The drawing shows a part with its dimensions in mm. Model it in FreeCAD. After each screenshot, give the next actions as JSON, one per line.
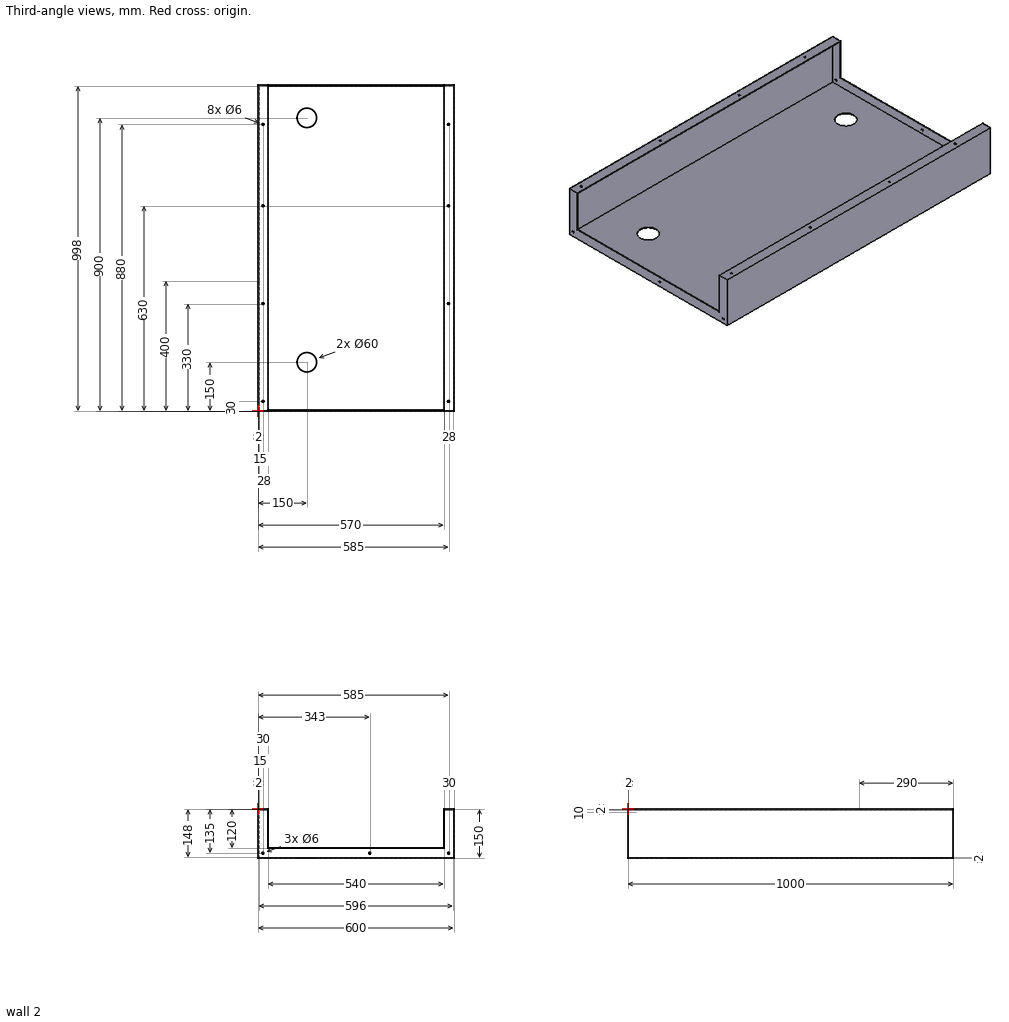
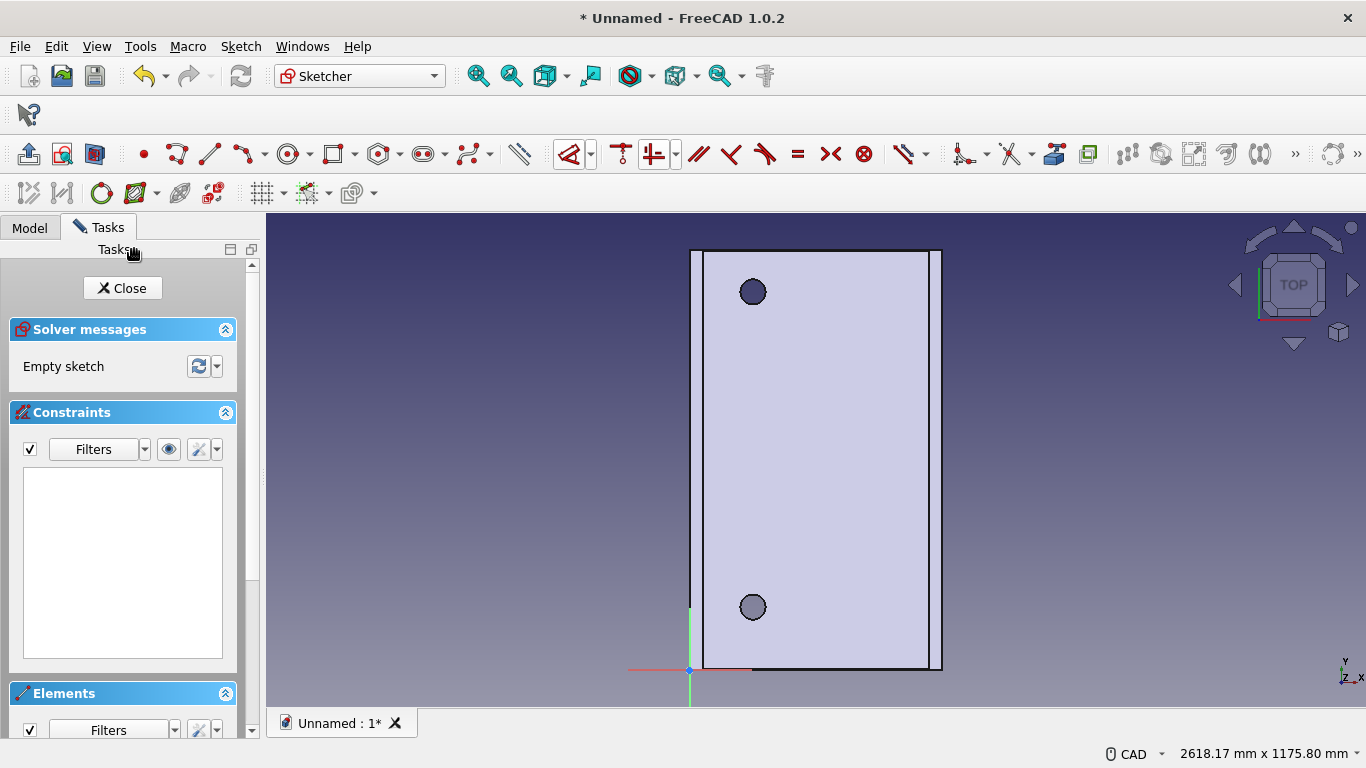
{"action": "scroll", "coordinate": [449, 349], "scroll_direction": "down", "scroll_amount": 1}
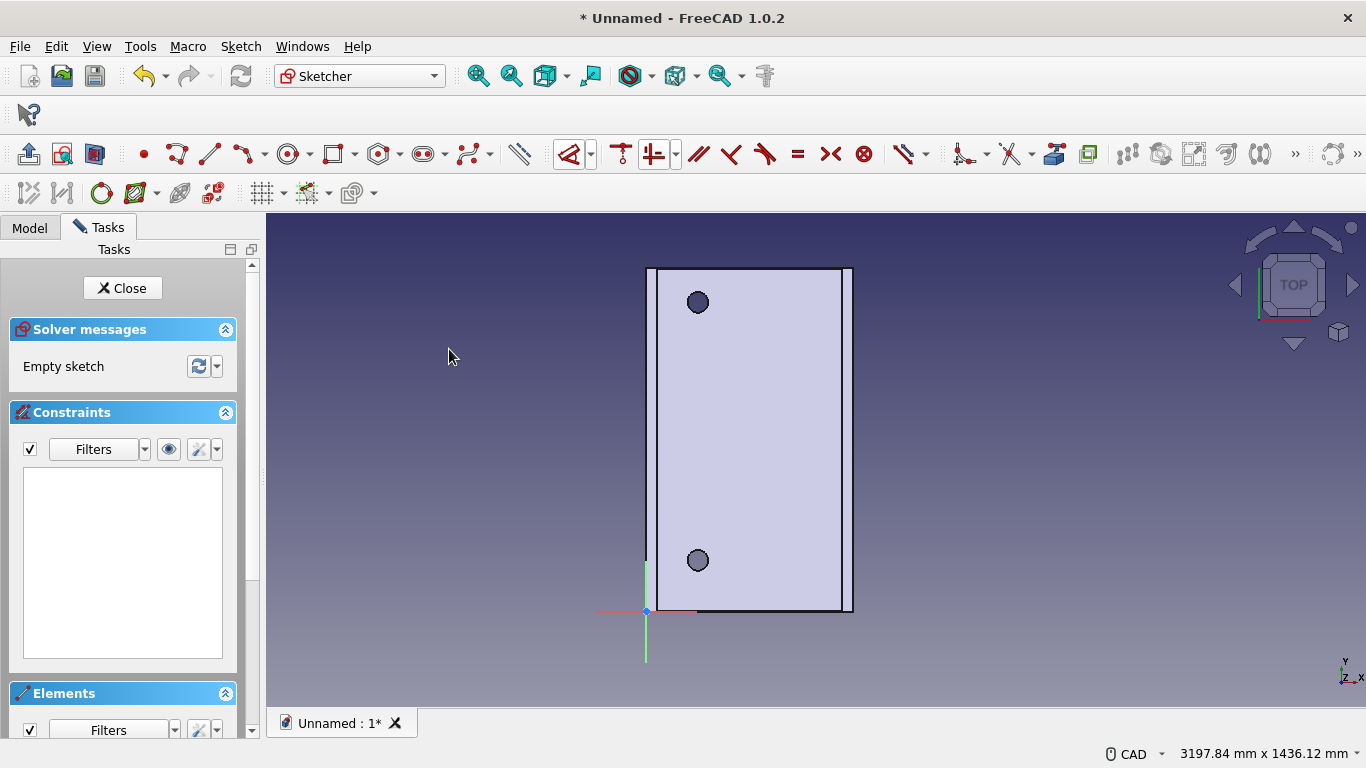
{"action": "left_click", "coordinate": [288, 154]}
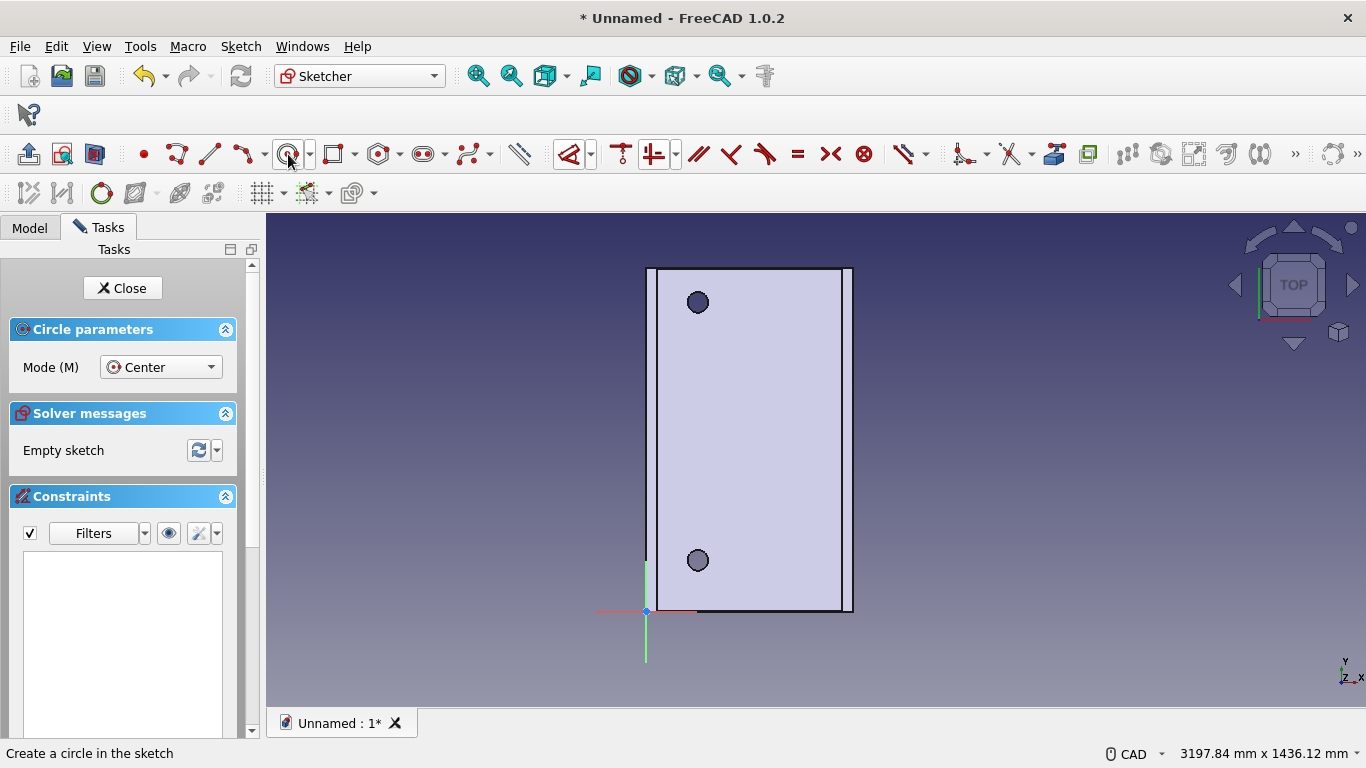
{"action": "scroll", "coordinate": [651, 309], "scroll_direction": "up", "scroll_amount": 16}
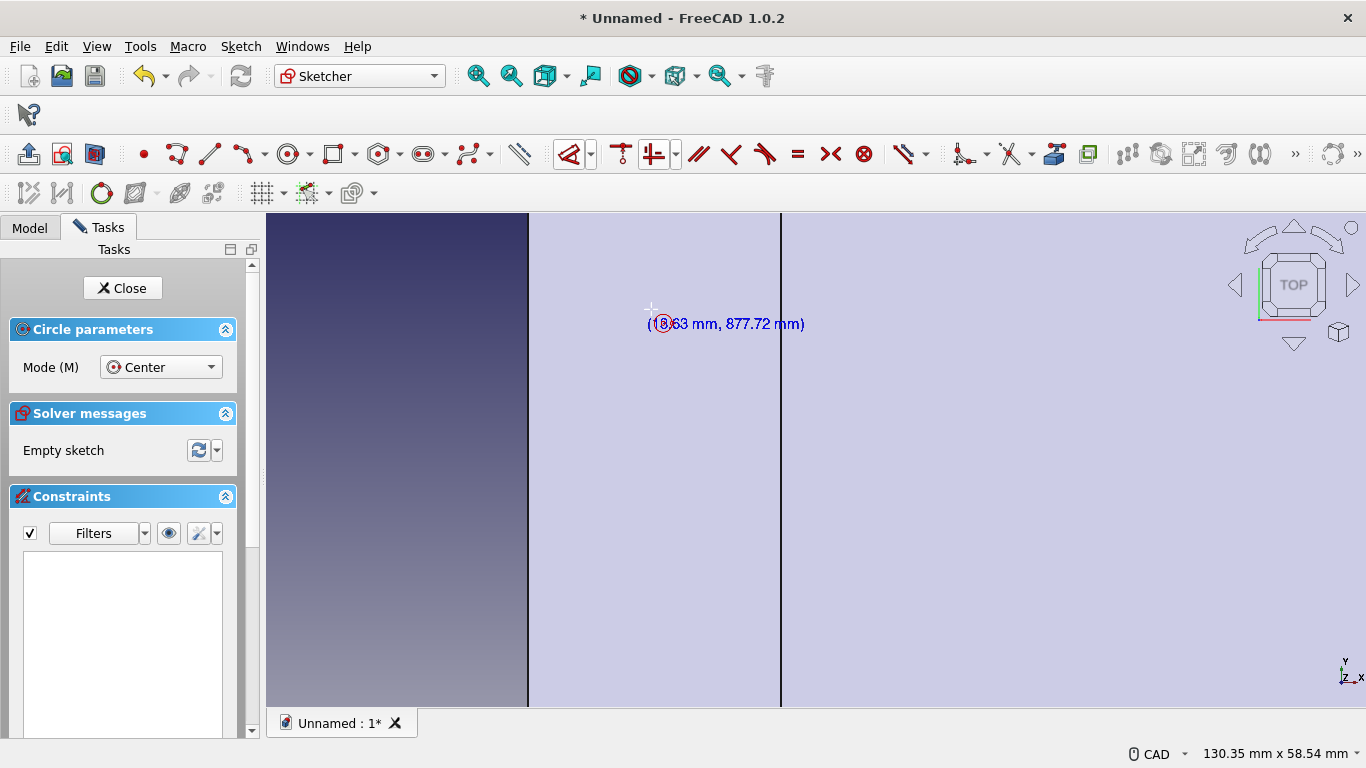
{"action": "scroll", "coordinate": [629, 274], "scroll_direction": "down", "scroll_amount": 15}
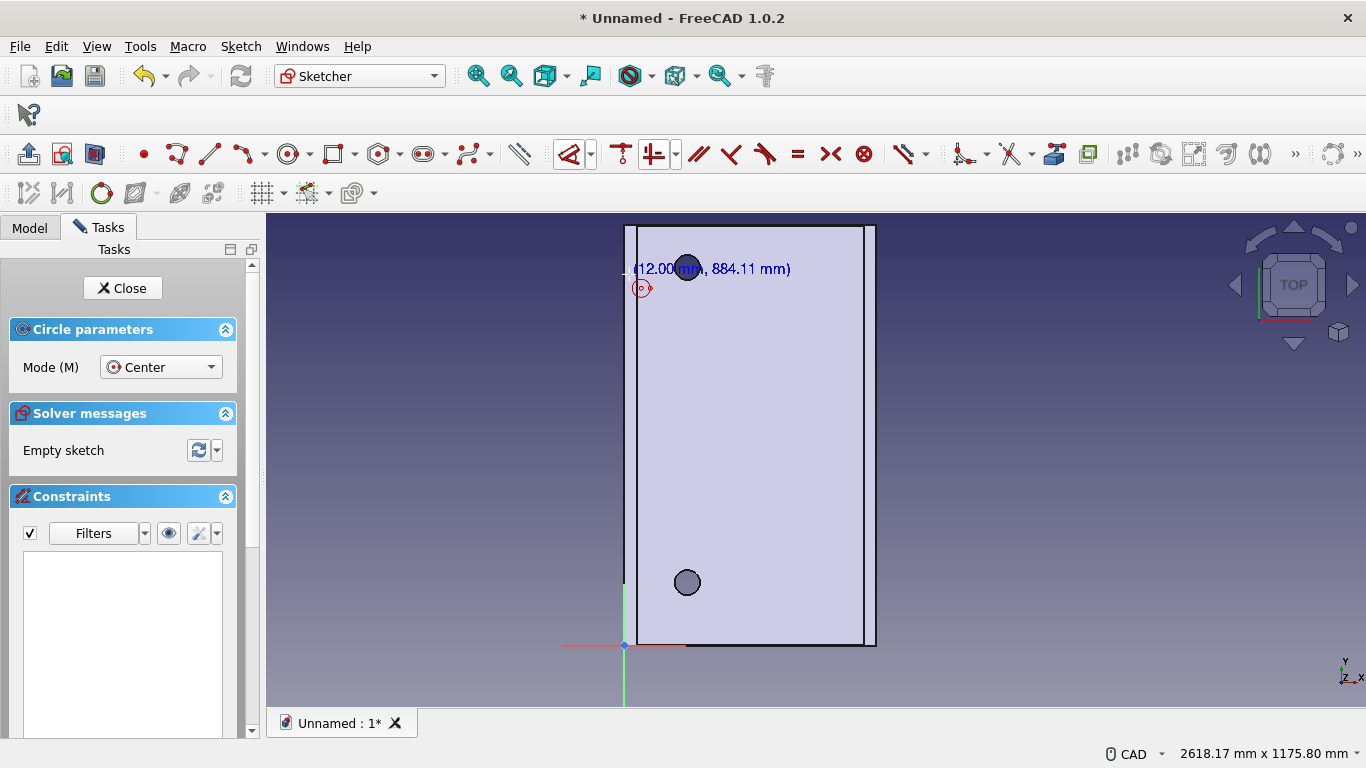
{"action": "scroll", "coordinate": [631, 276], "scroll_direction": "up", "scroll_amount": 5}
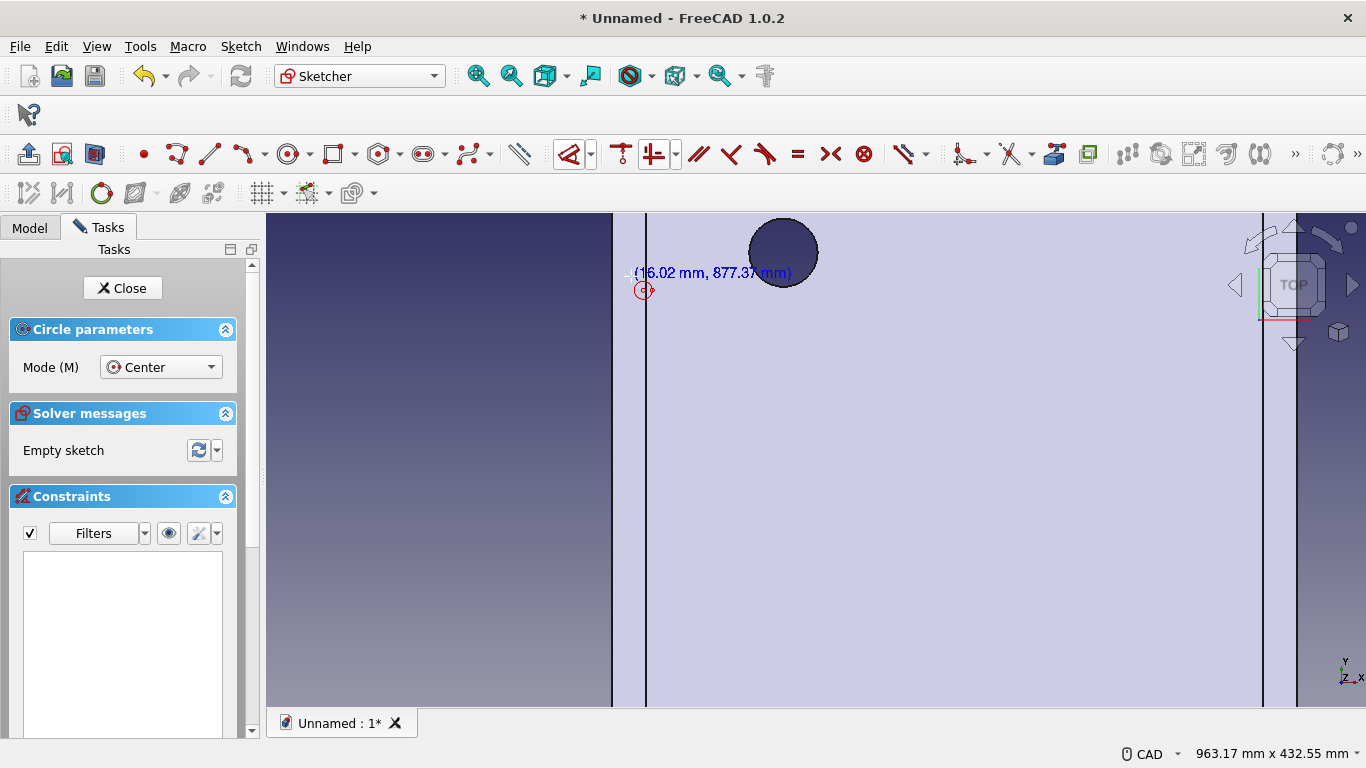
{"action": "left_click", "coordinate": [629, 275]}
{"action": "mouse_move", "coordinate": [632, 273]}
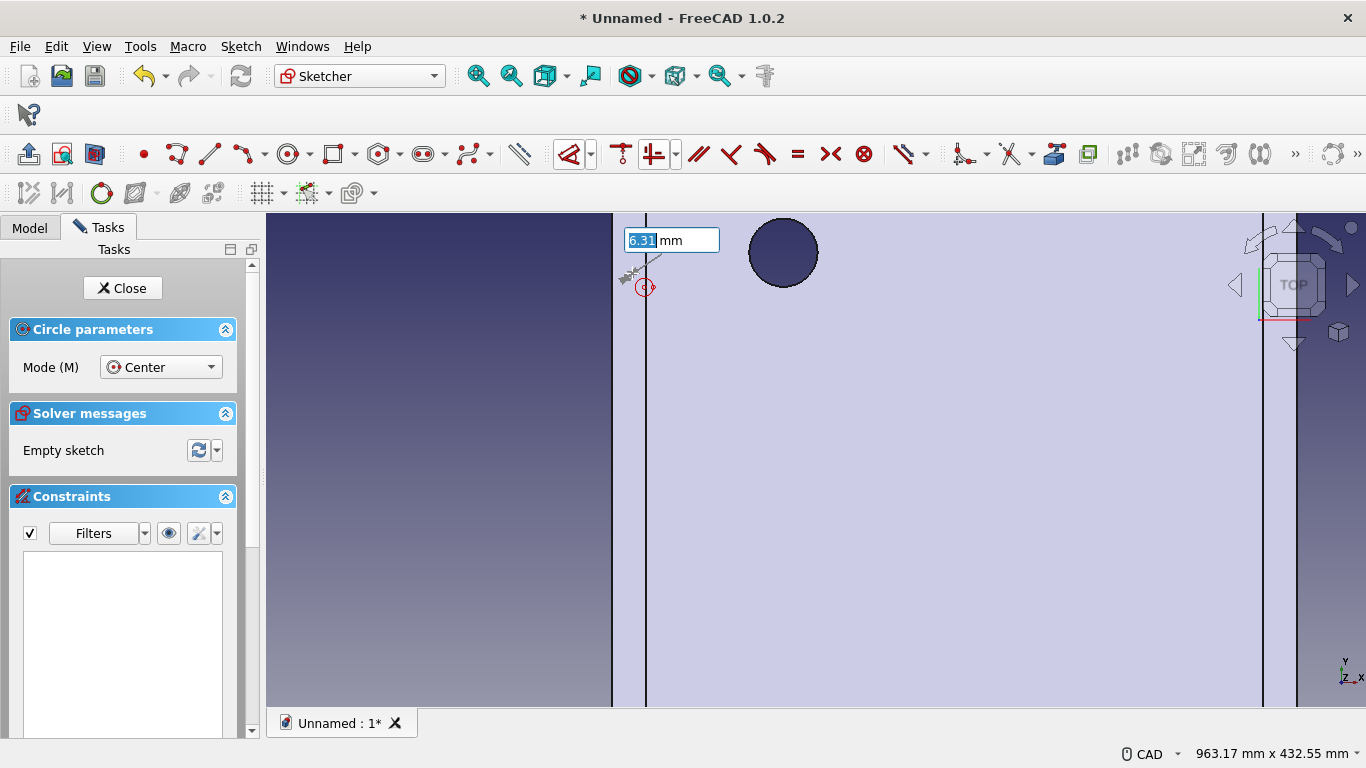
{"action": "type", "text": "6"}
{"action": "key", "text": "Return"}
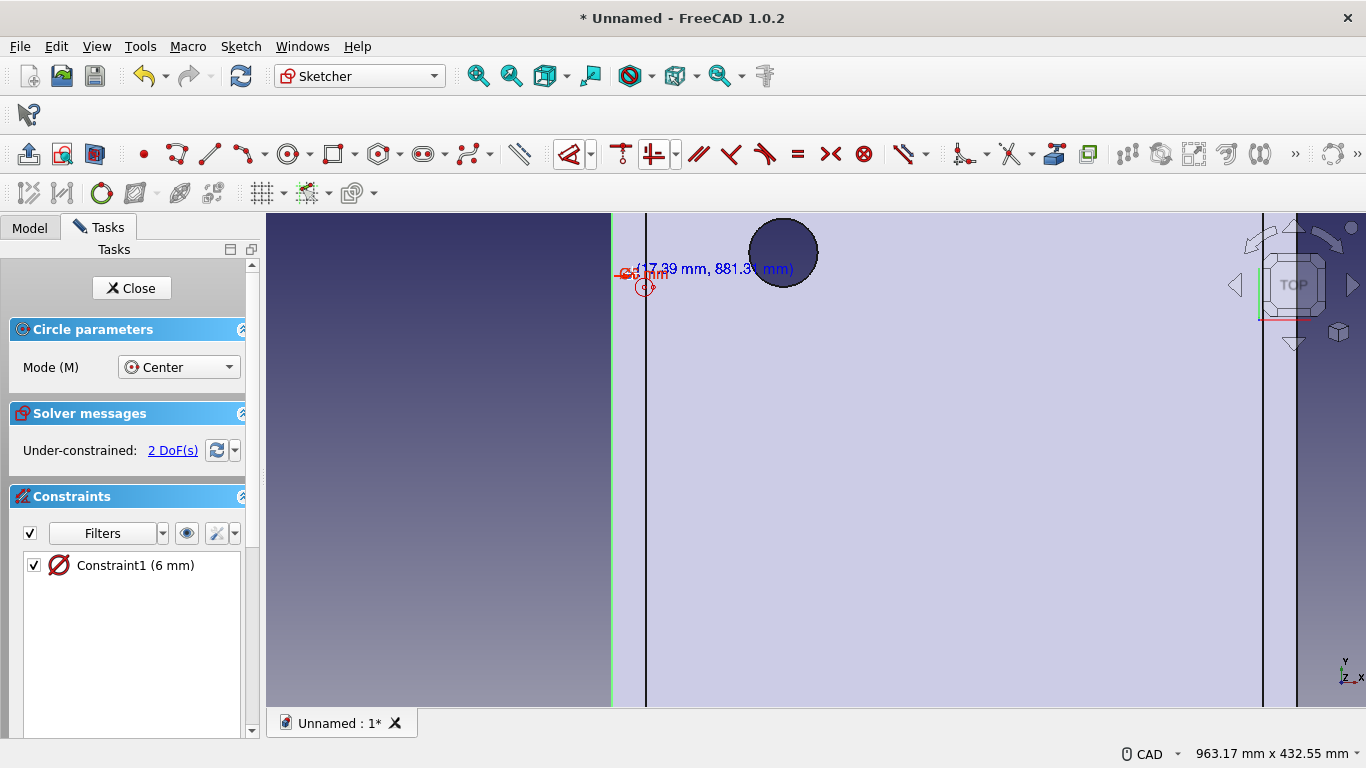
{"action": "scroll", "coordinate": [661, 324], "scroll_direction": "down", "scroll_amount": 6}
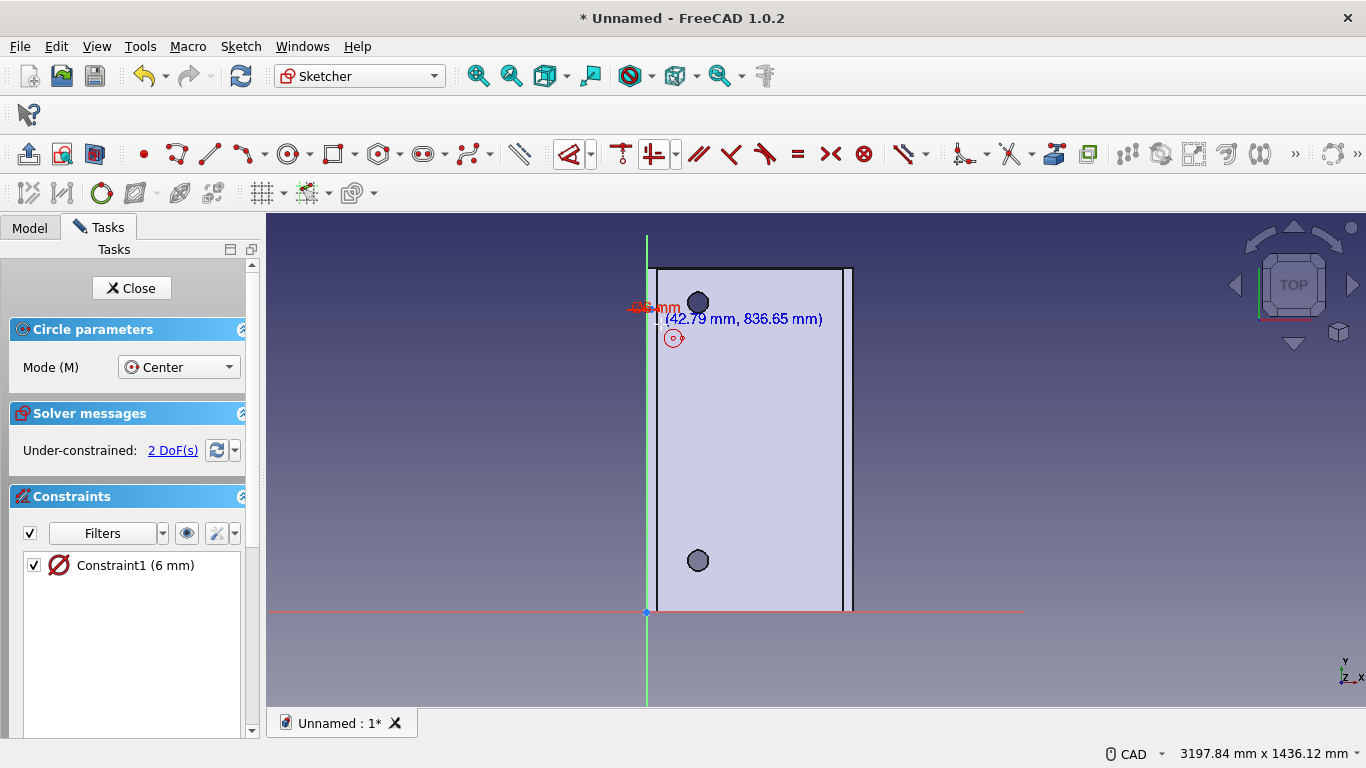
{"action": "scroll", "coordinate": [652, 602], "scroll_direction": "up", "scroll_amount": 16}